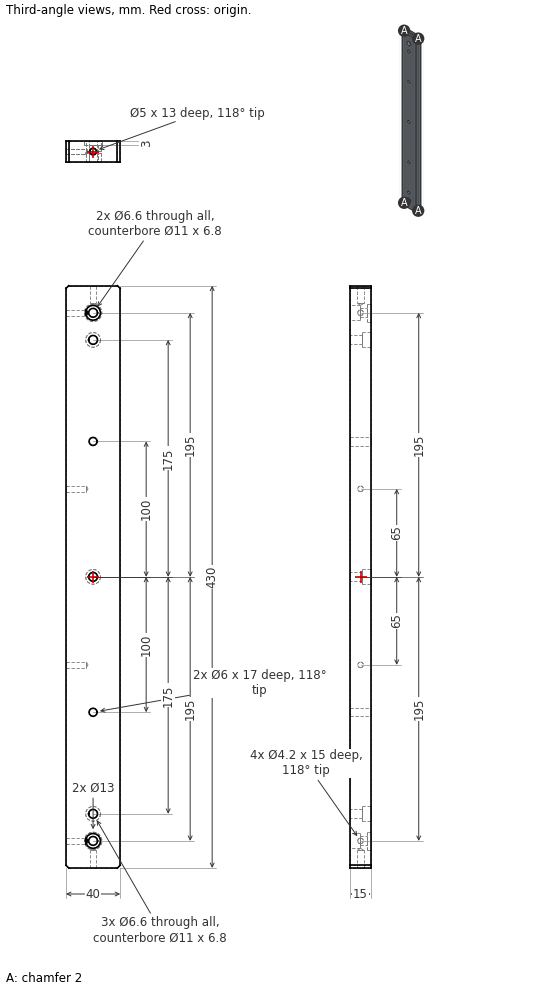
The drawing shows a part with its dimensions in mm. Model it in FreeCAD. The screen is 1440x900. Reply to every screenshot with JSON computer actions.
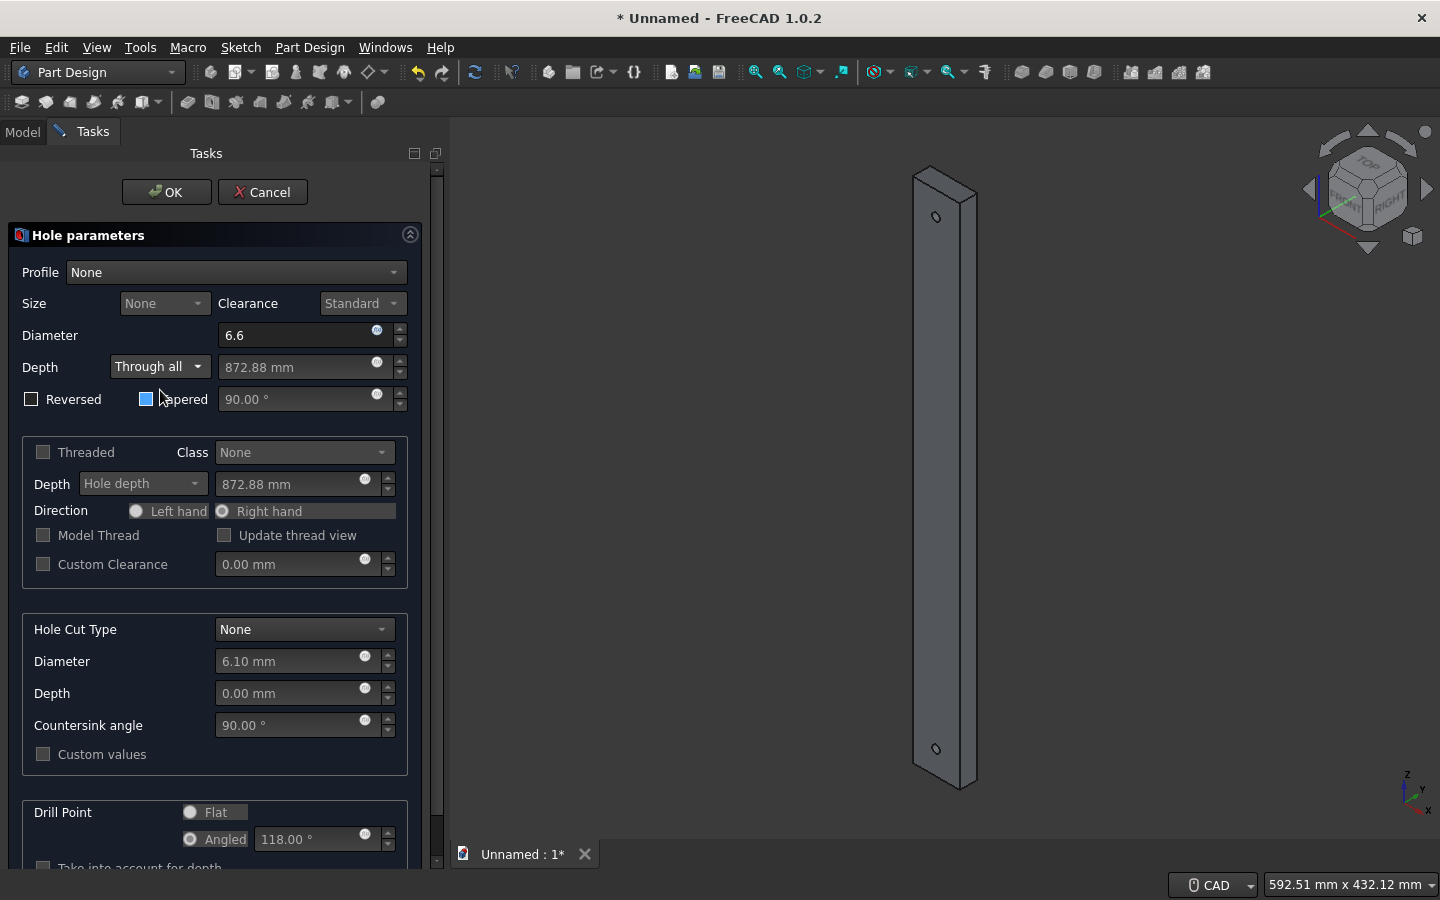
{"action": "left_click", "coordinate": [306, 630]}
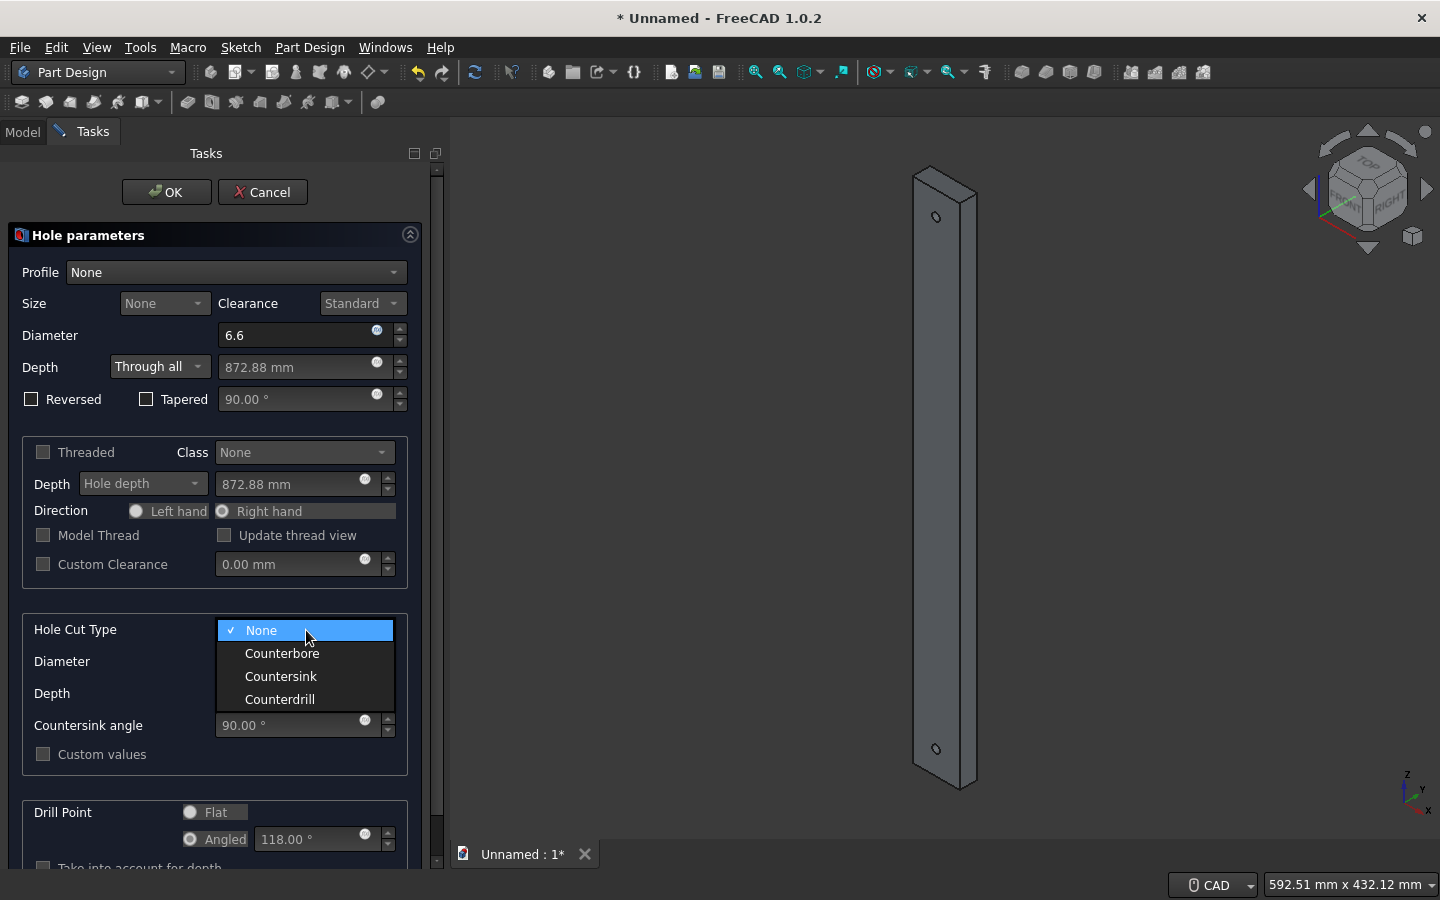
{"action": "left_click", "coordinate": [304, 654]}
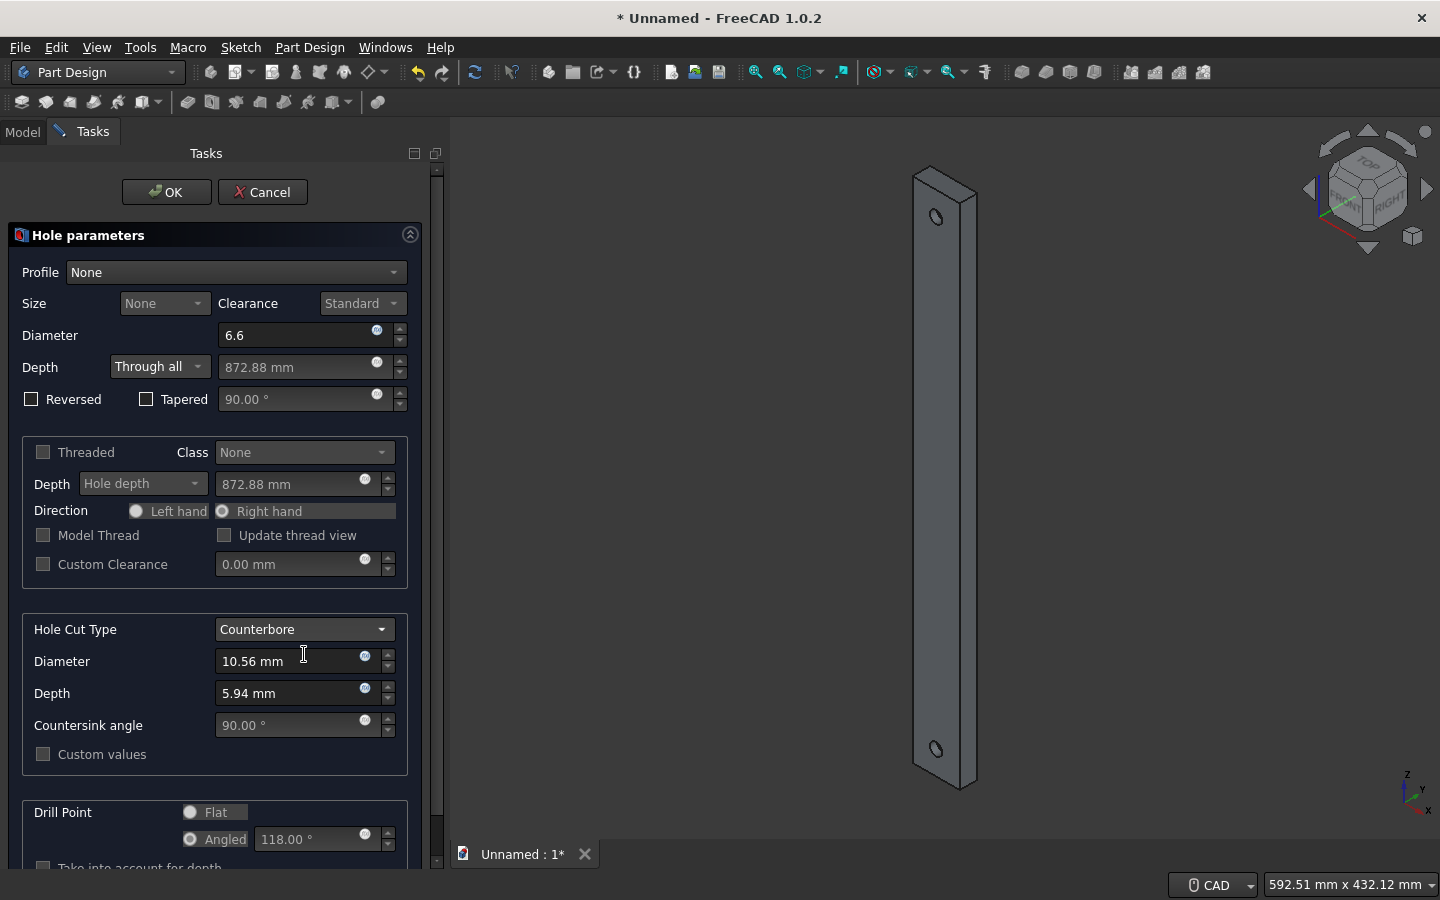
{"action": "triple_click", "coordinate": [298, 661]}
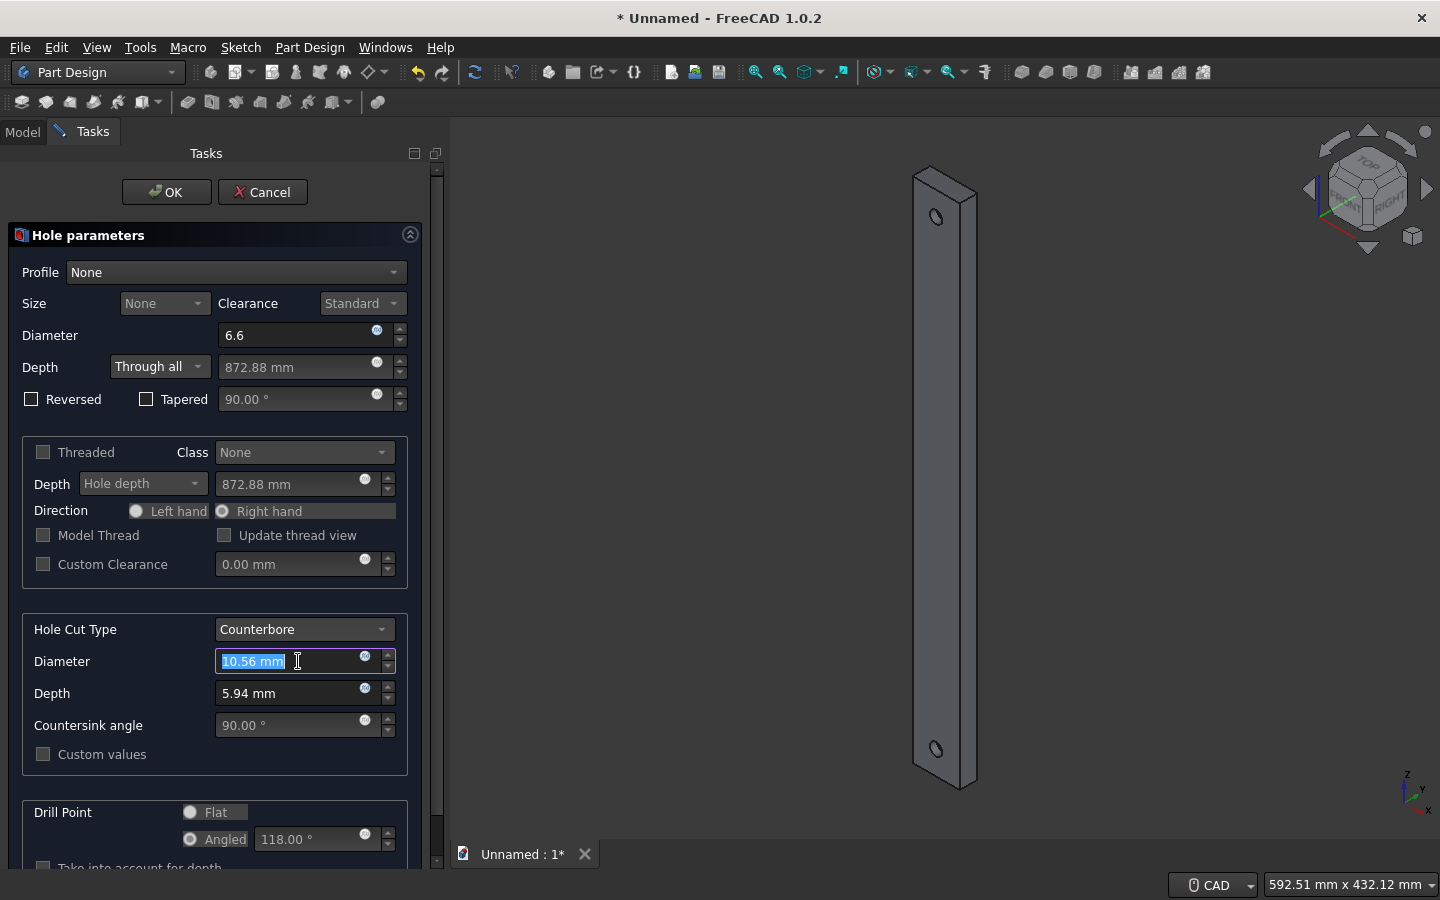
{"action": "type", "text": "11"}
{"action": "key", "text": "Tab"}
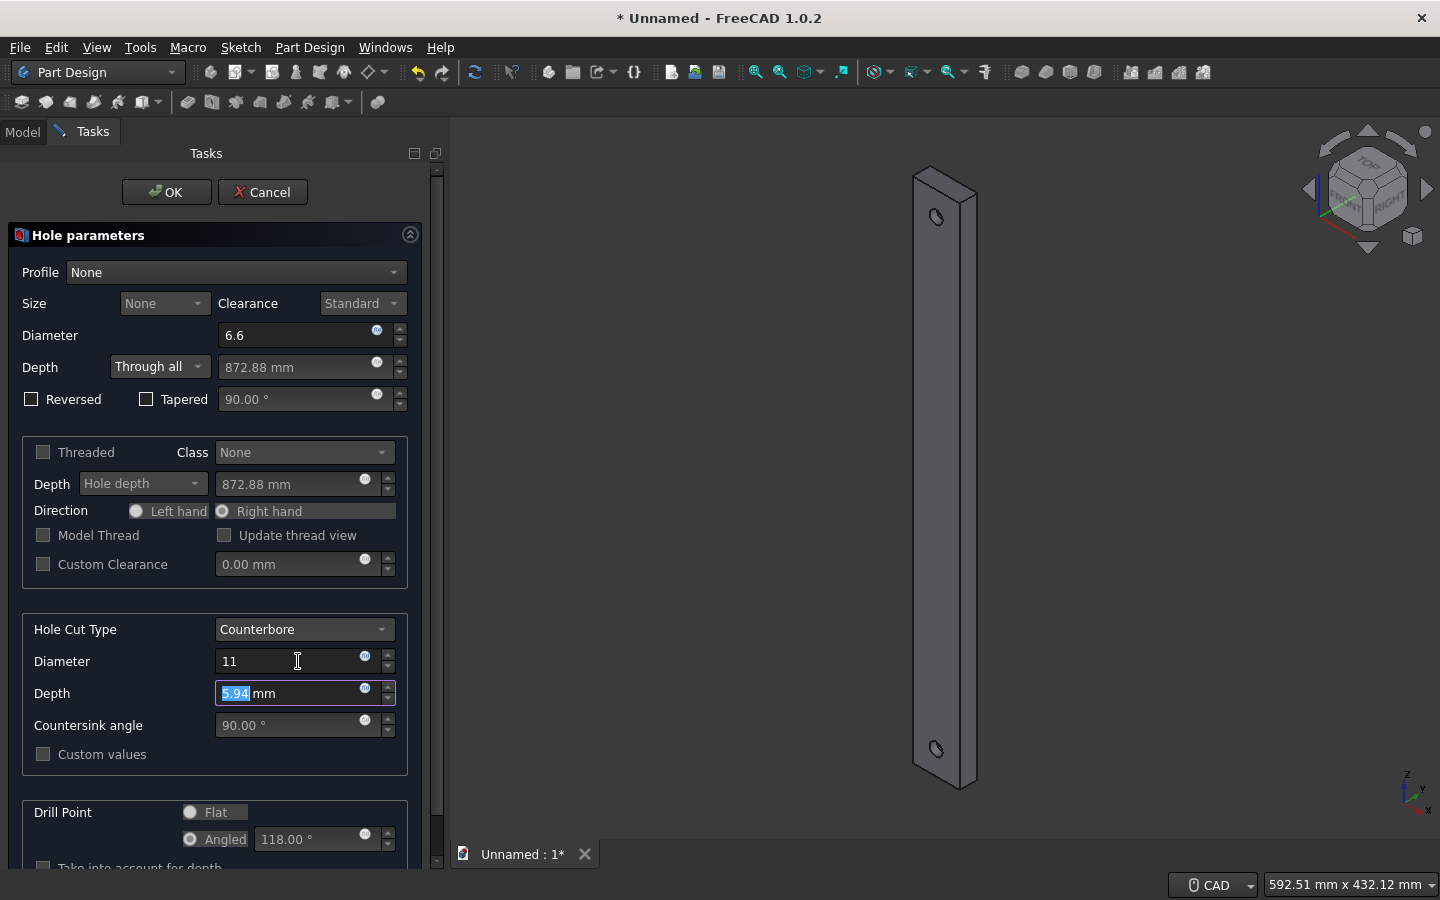
{"action": "type", "text": "6.8"}
{"action": "key", "text": "Tab"}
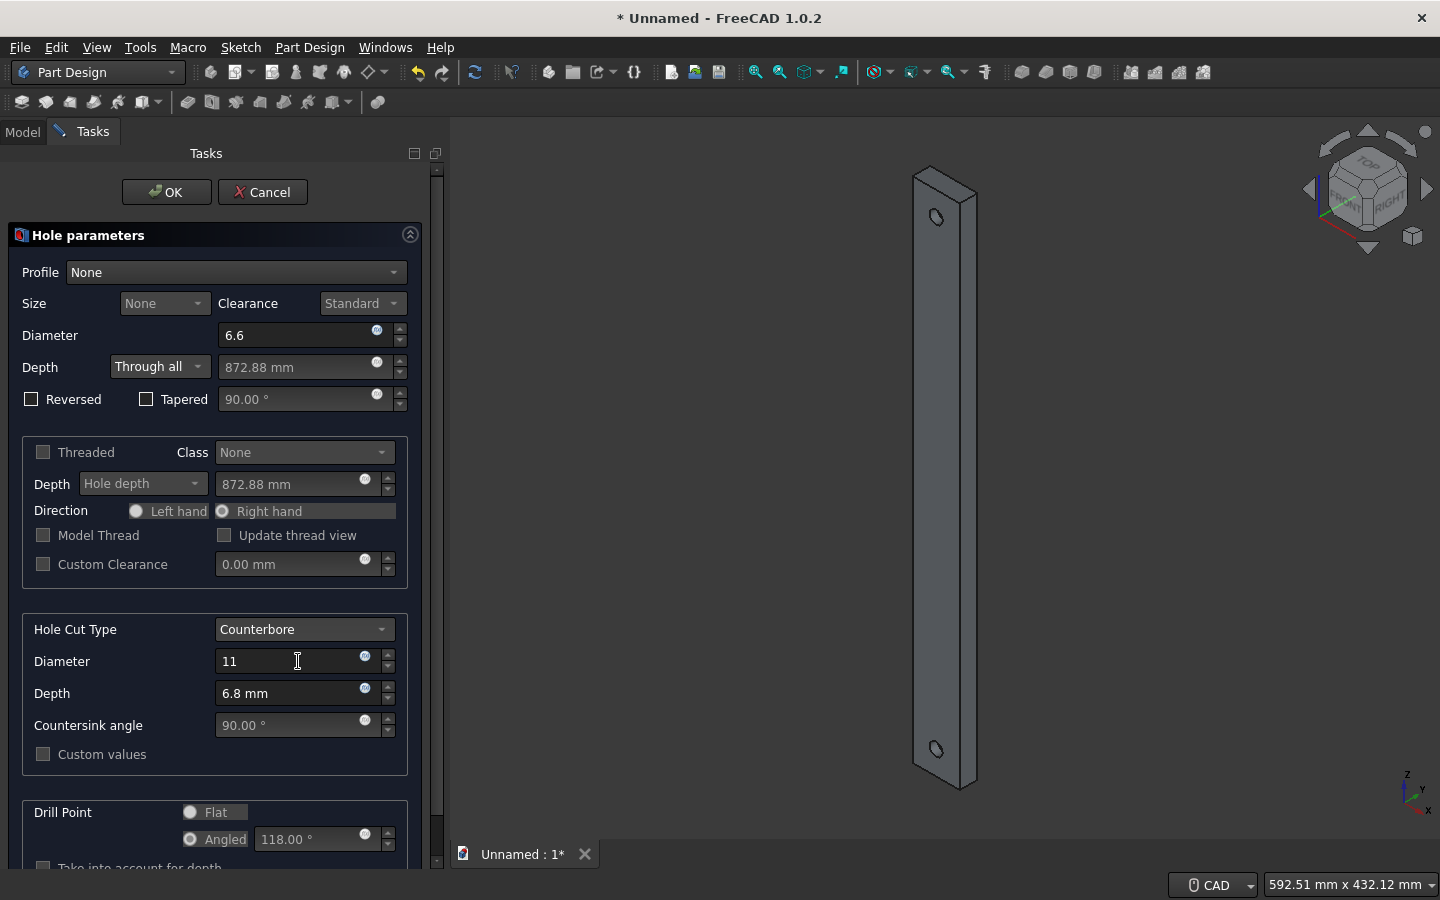
{"action": "left_click", "coordinate": [167, 192]}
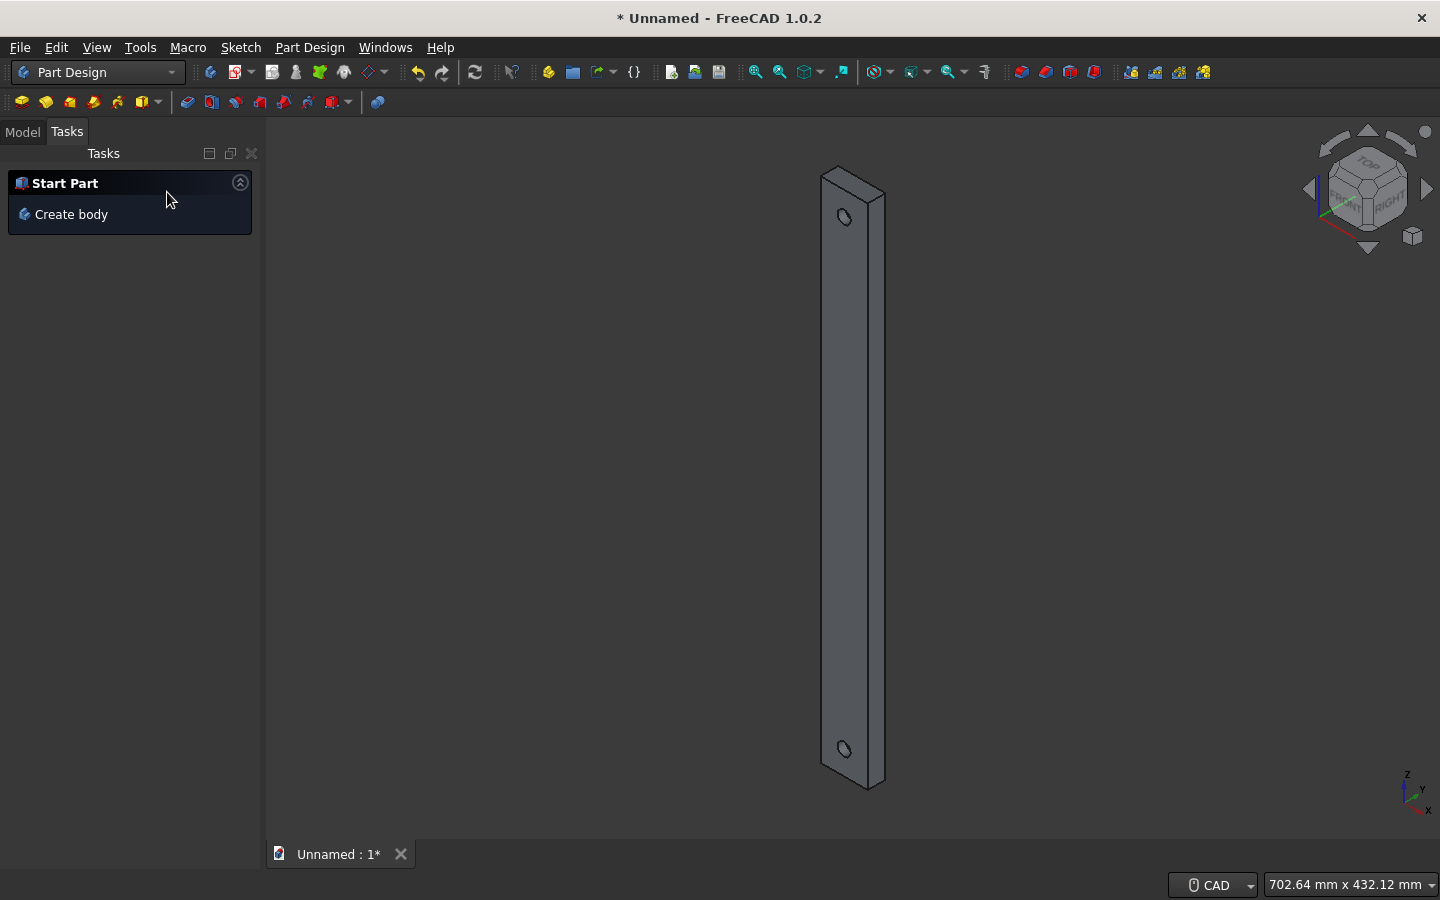
{"action": "key", "text": "6"}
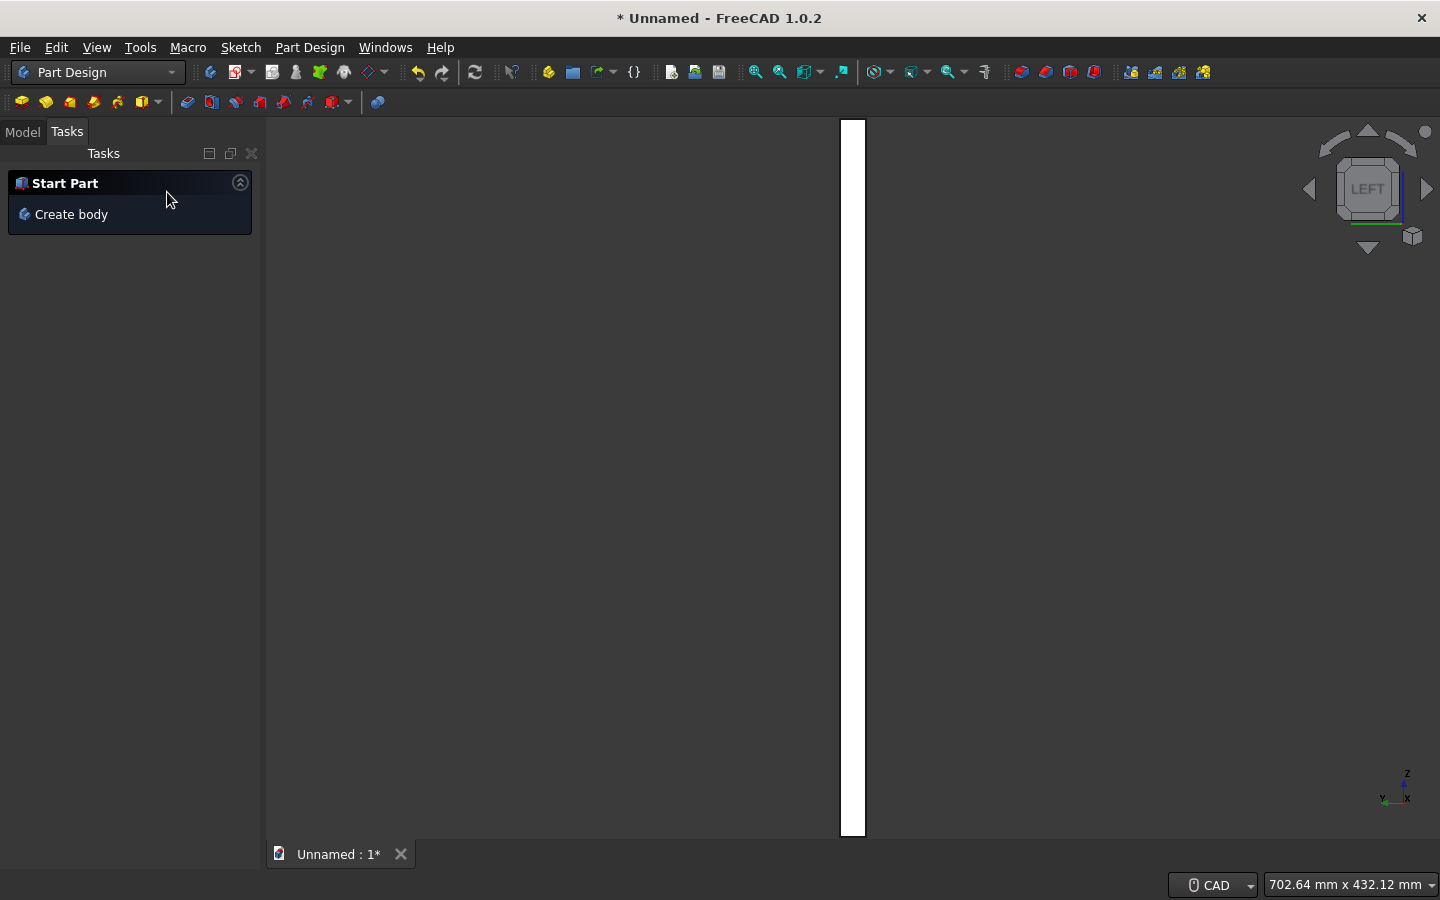
{"action": "left_click", "coordinate": [853, 272]}